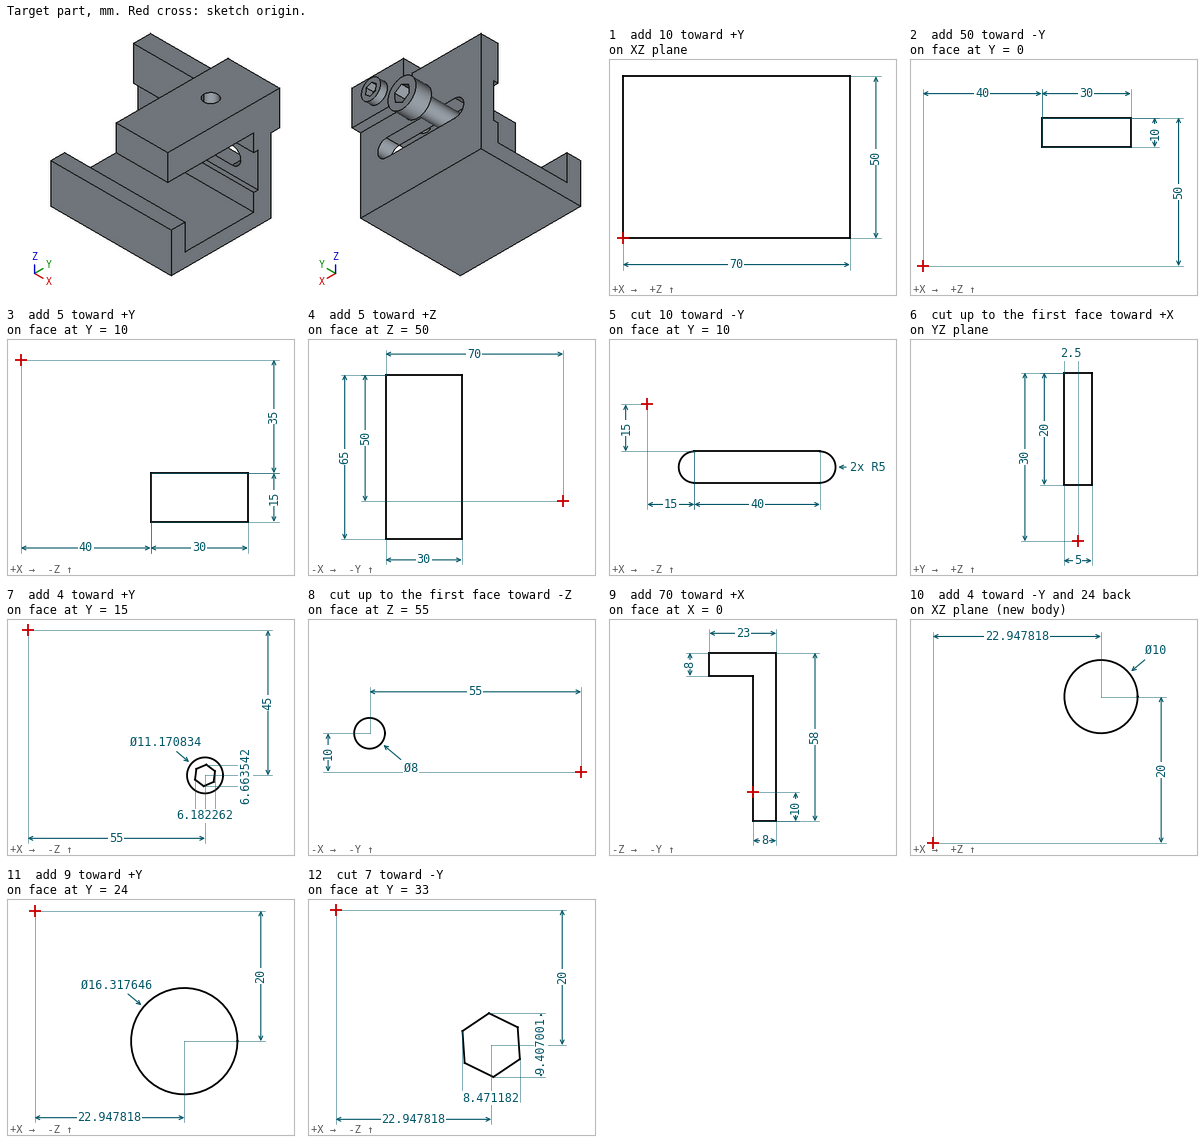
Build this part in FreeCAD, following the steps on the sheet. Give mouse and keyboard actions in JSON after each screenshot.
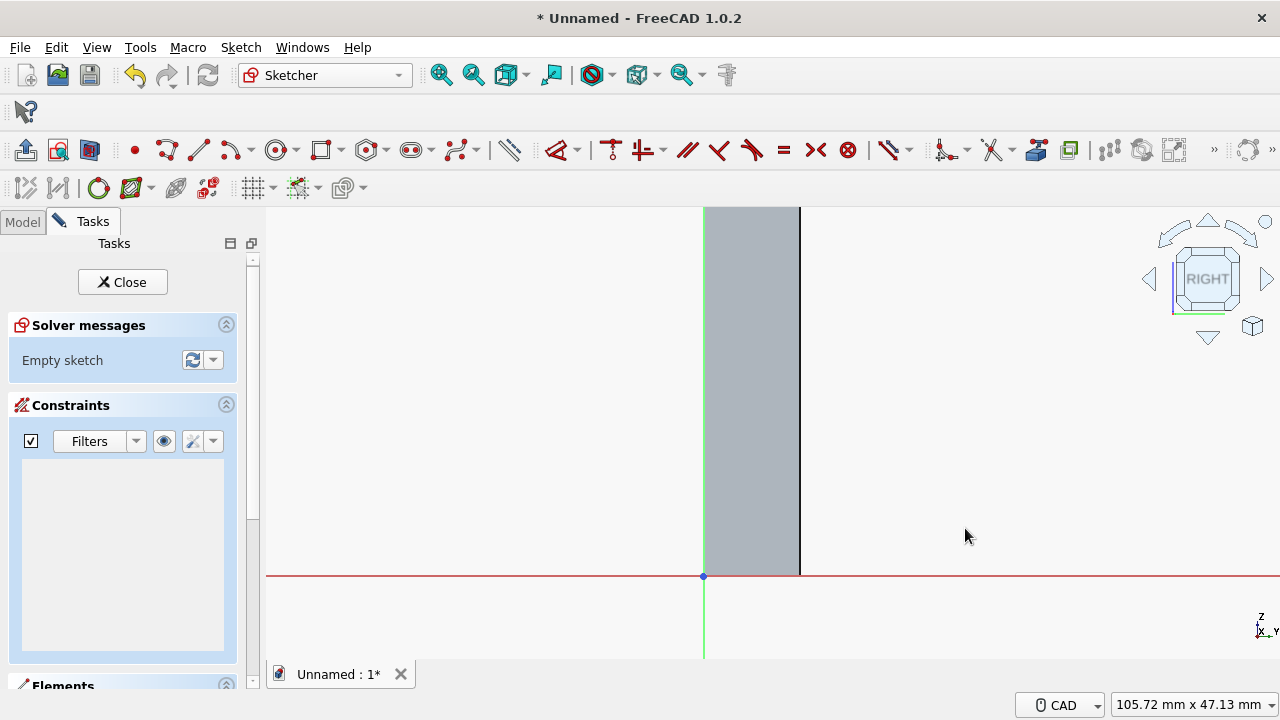
{"action": "left_click", "coordinate": [322, 150]}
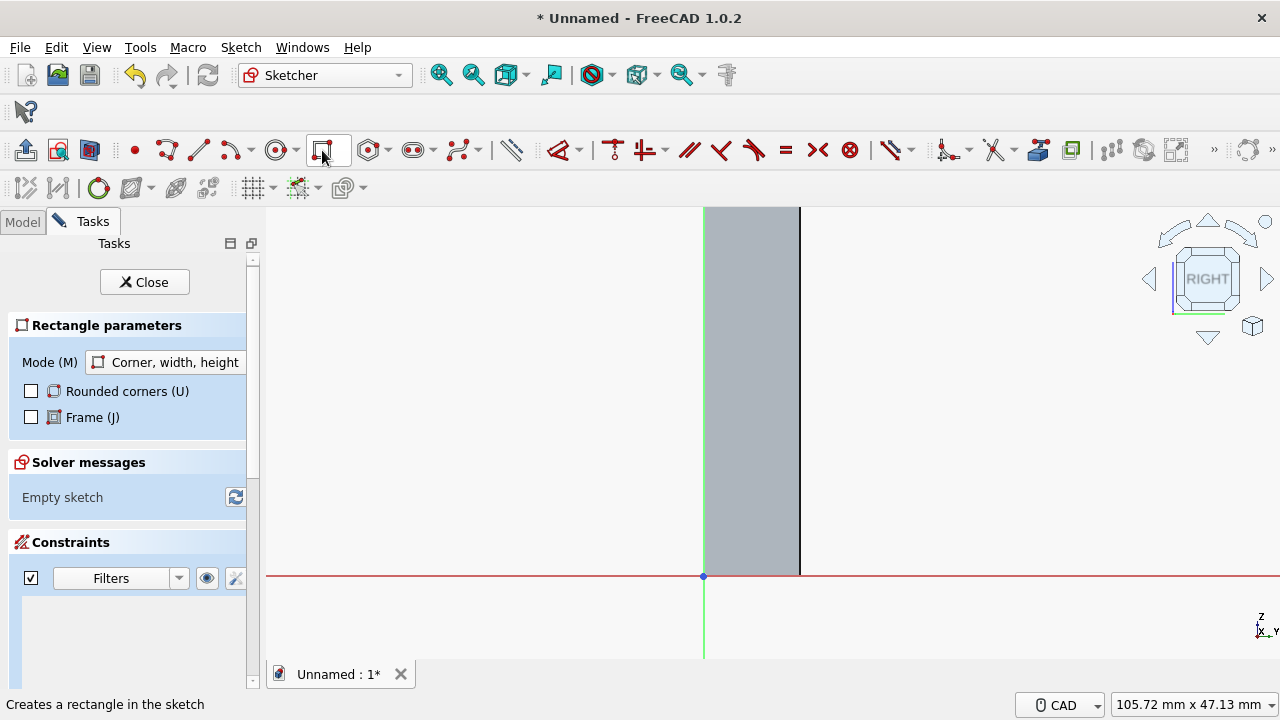
{"action": "left_click", "coordinate": [680, 289]}
{"action": "left_click", "coordinate": [728, 480]}
{"action": "key", "text": "Escape"}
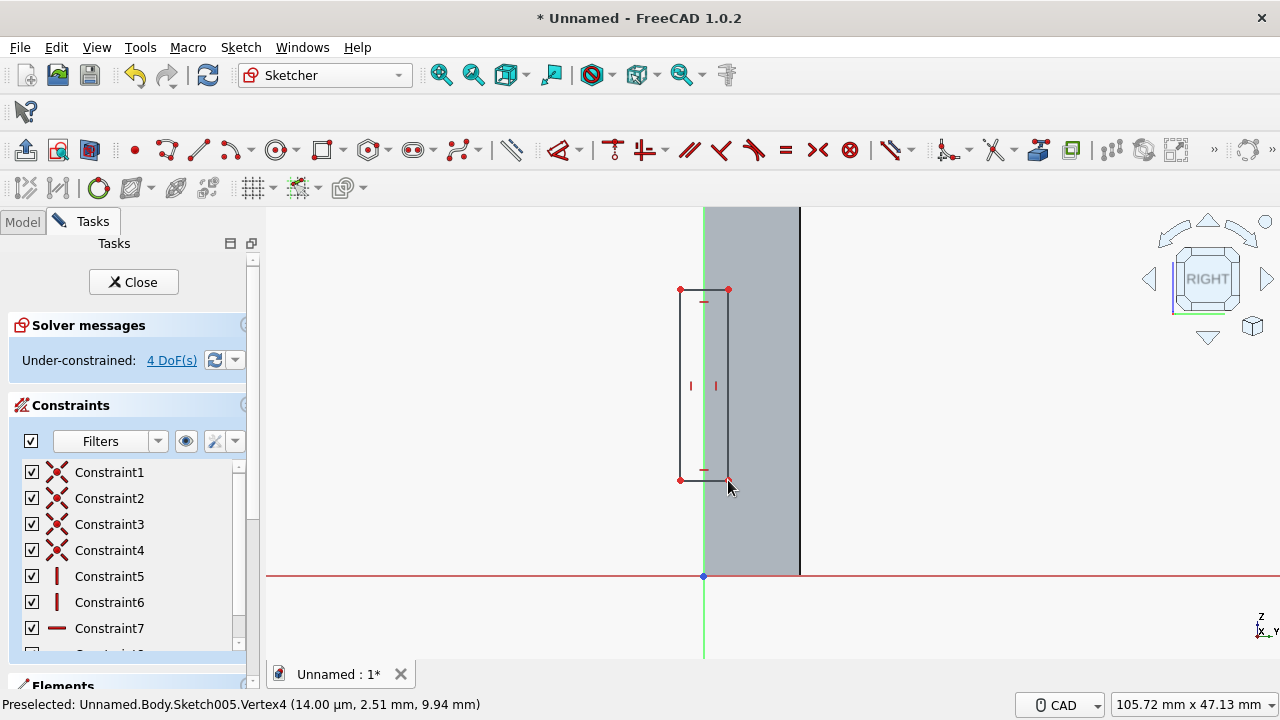
{"action": "left_click", "coordinate": [558, 150]}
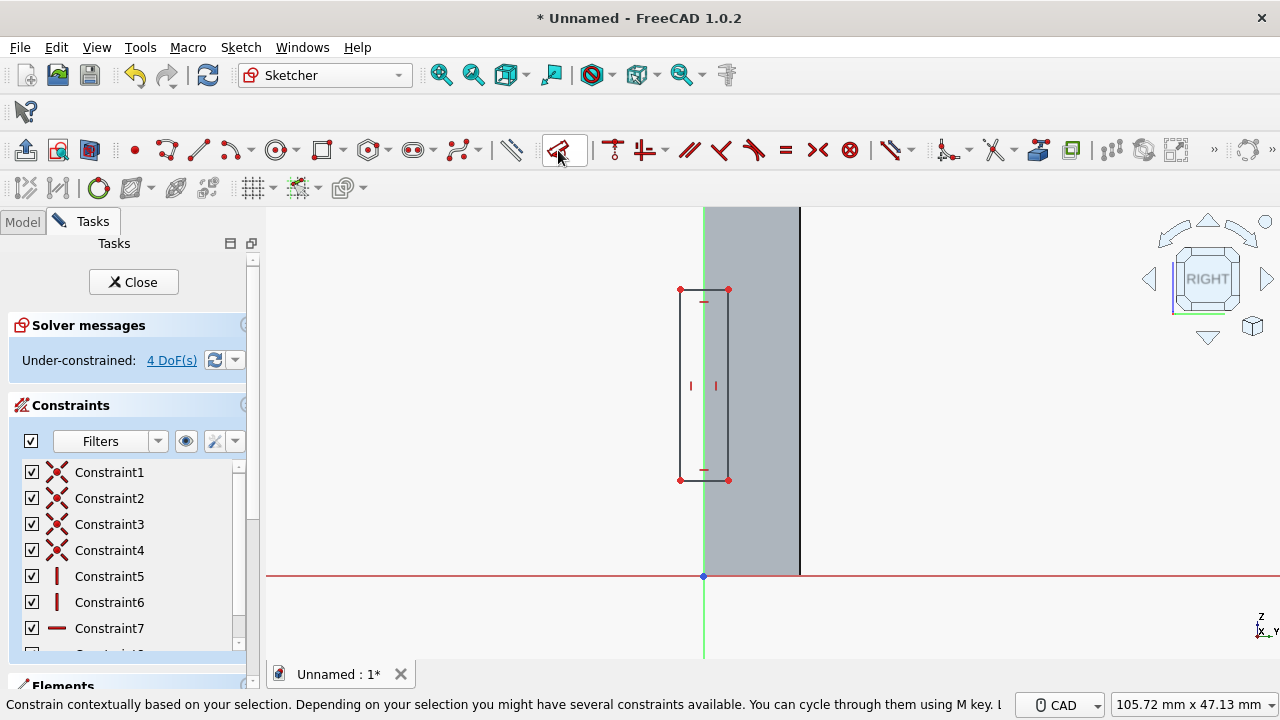
{"action": "scroll", "coordinate": [694, 481], "scroll_direction": "up", "scroll_amount": 2}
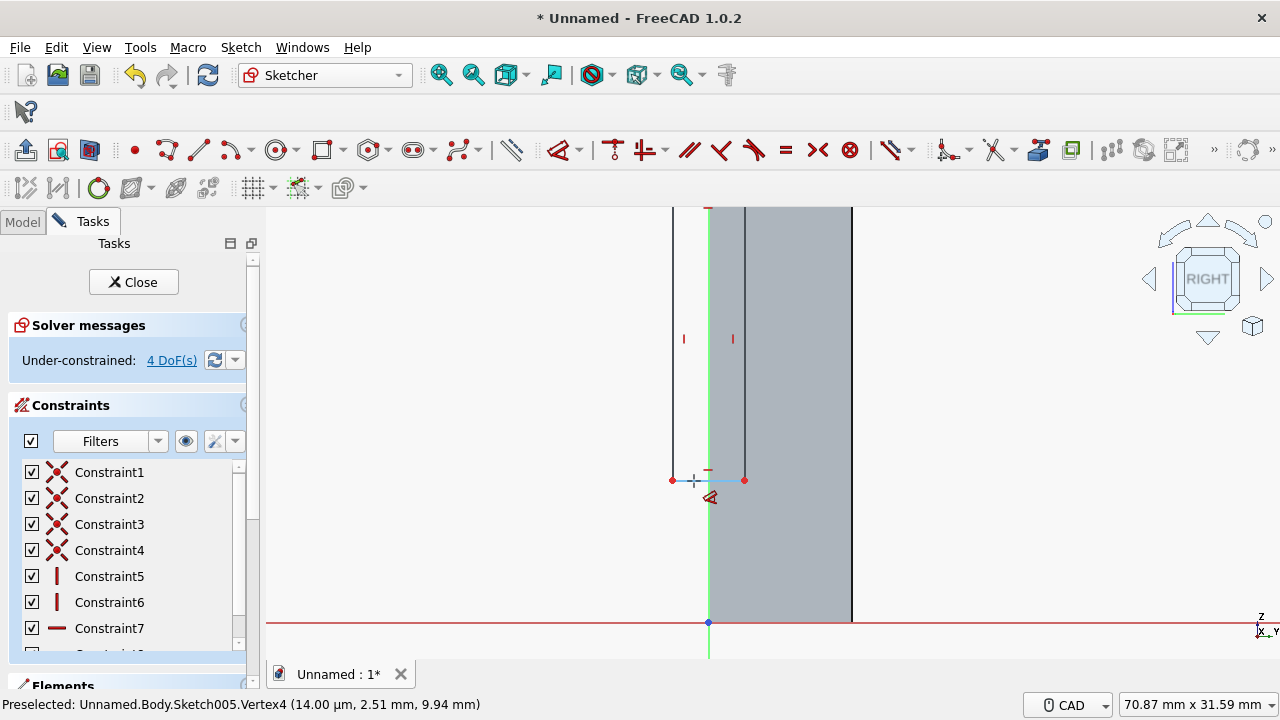
{"action": "left_click", "coordinate": [694, 481]}
{"action": "left_click", "coordinate": [692, 515]}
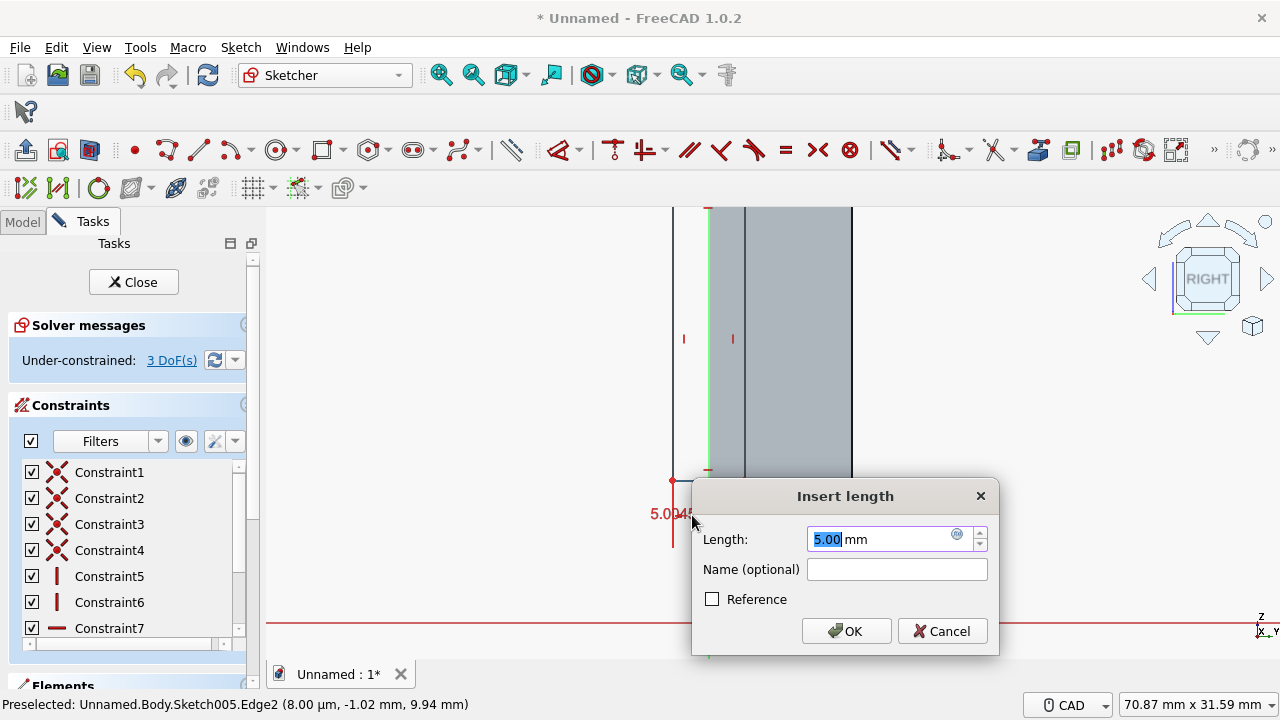
{"action": "type", "text": "5"}
{"action": "key", "text": "Return"}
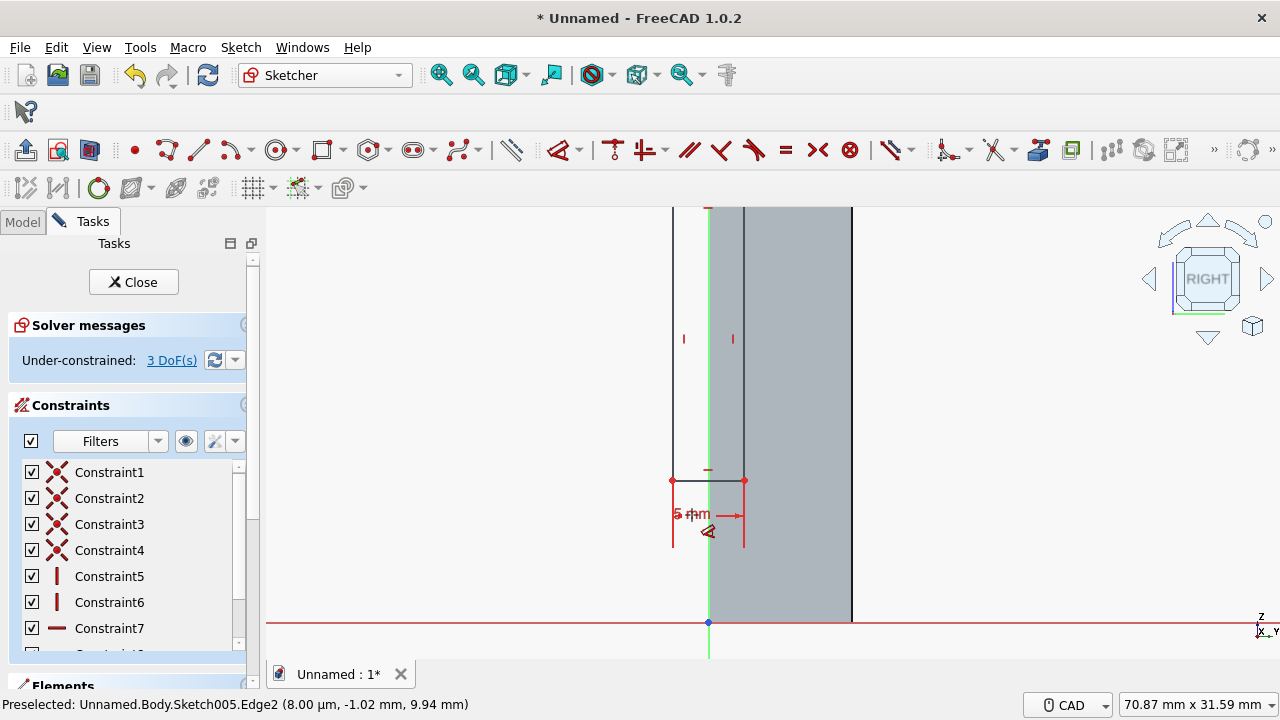
{"action": "left_click", "coordinate": [673, 281]}
{"action": "left_click", "coordinate": [639, 358]}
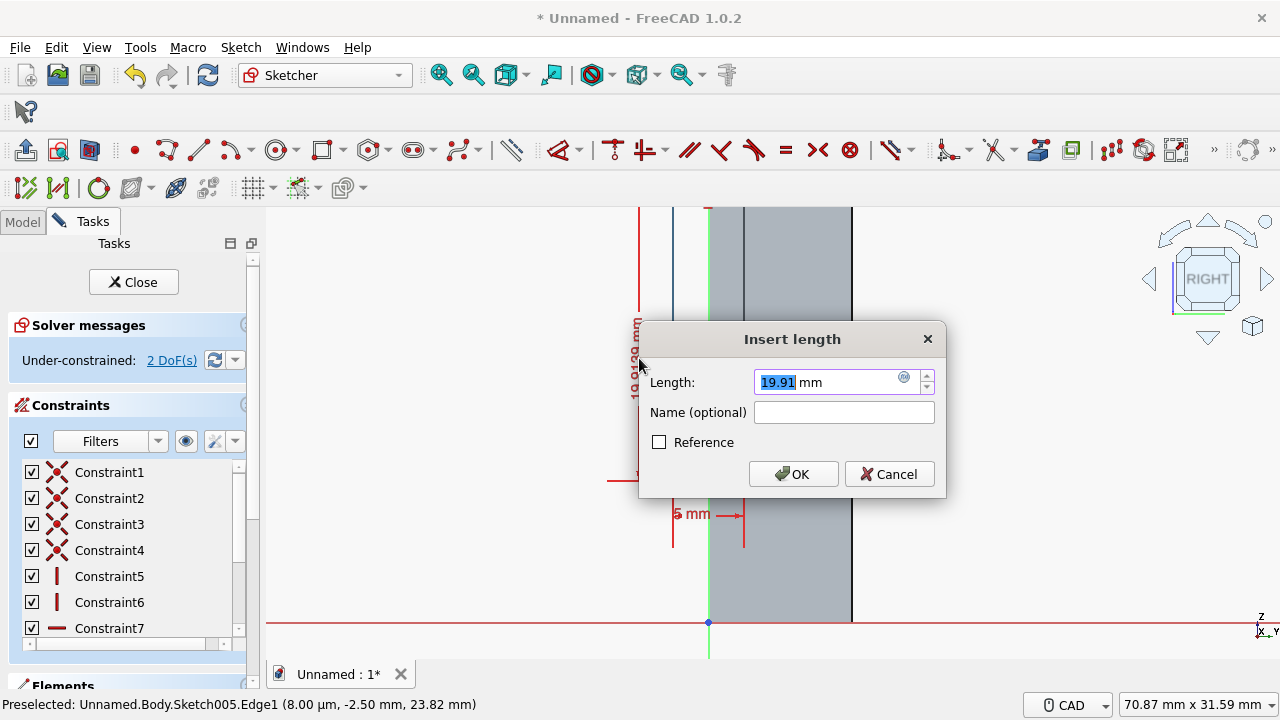
{"action": "type", "text": "20"}
{"action": "key", "text": "Return"}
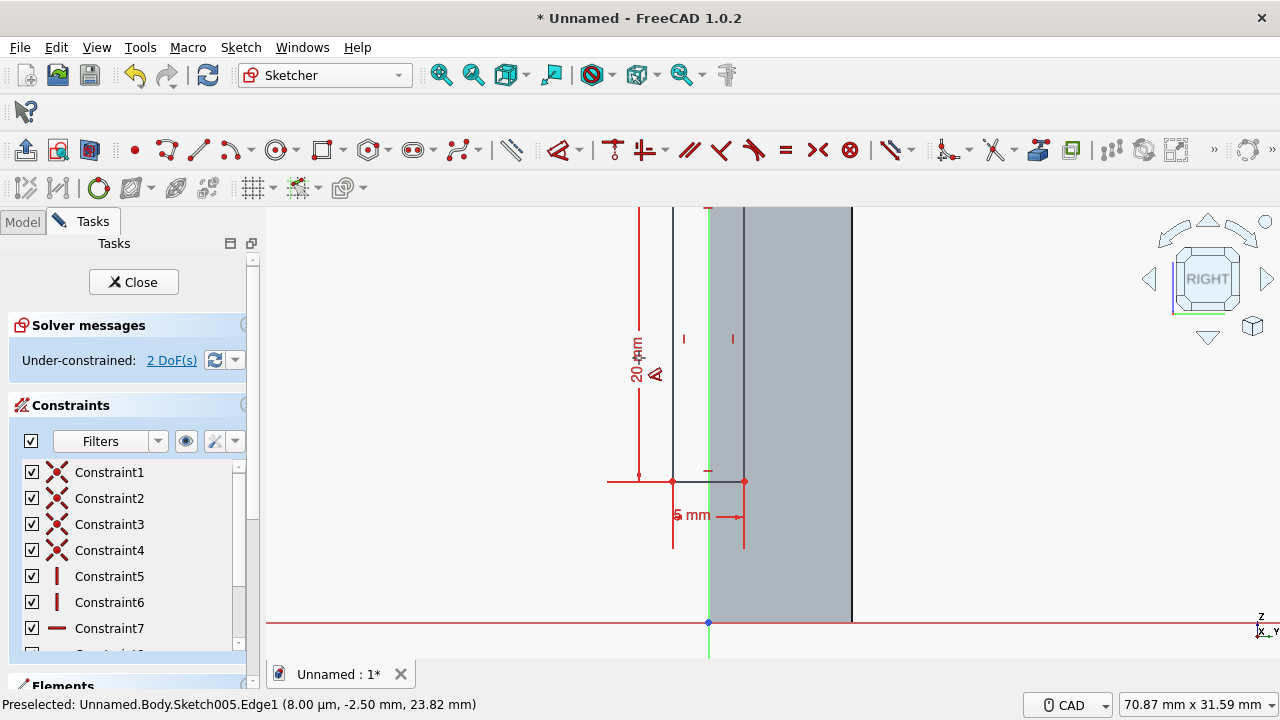
{"action": "scroll", "coordinate": [696, 483], "scroll_direction": "down", "scroll_amount": 2}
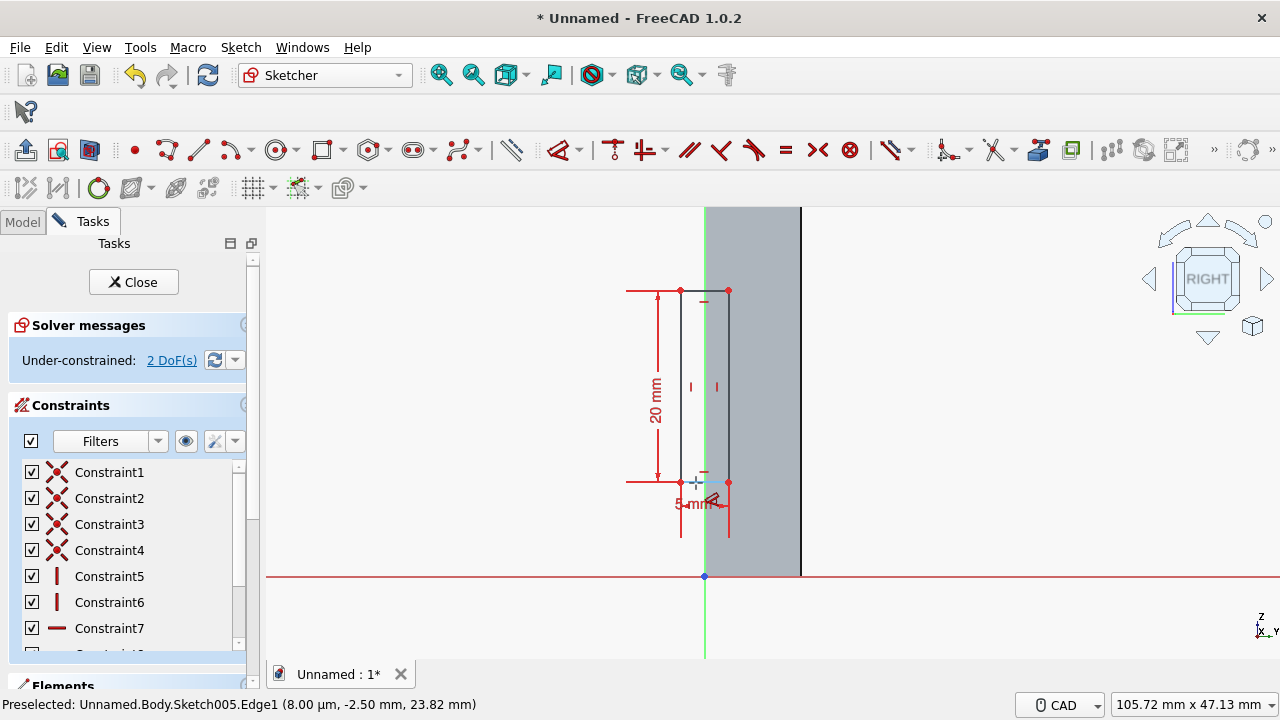
{"action": "left_click", "coordinate": [681, 291]}
{"action": "left_click", "coordinate": [647, 434]}